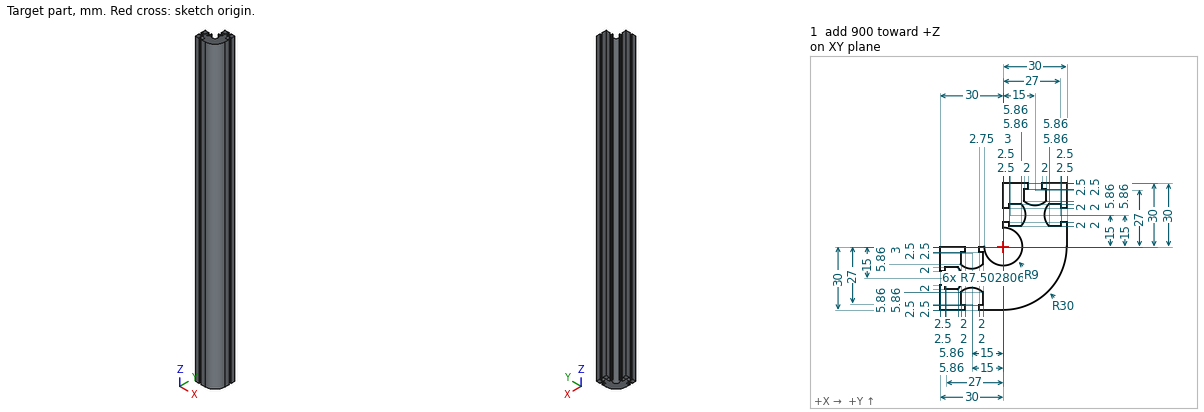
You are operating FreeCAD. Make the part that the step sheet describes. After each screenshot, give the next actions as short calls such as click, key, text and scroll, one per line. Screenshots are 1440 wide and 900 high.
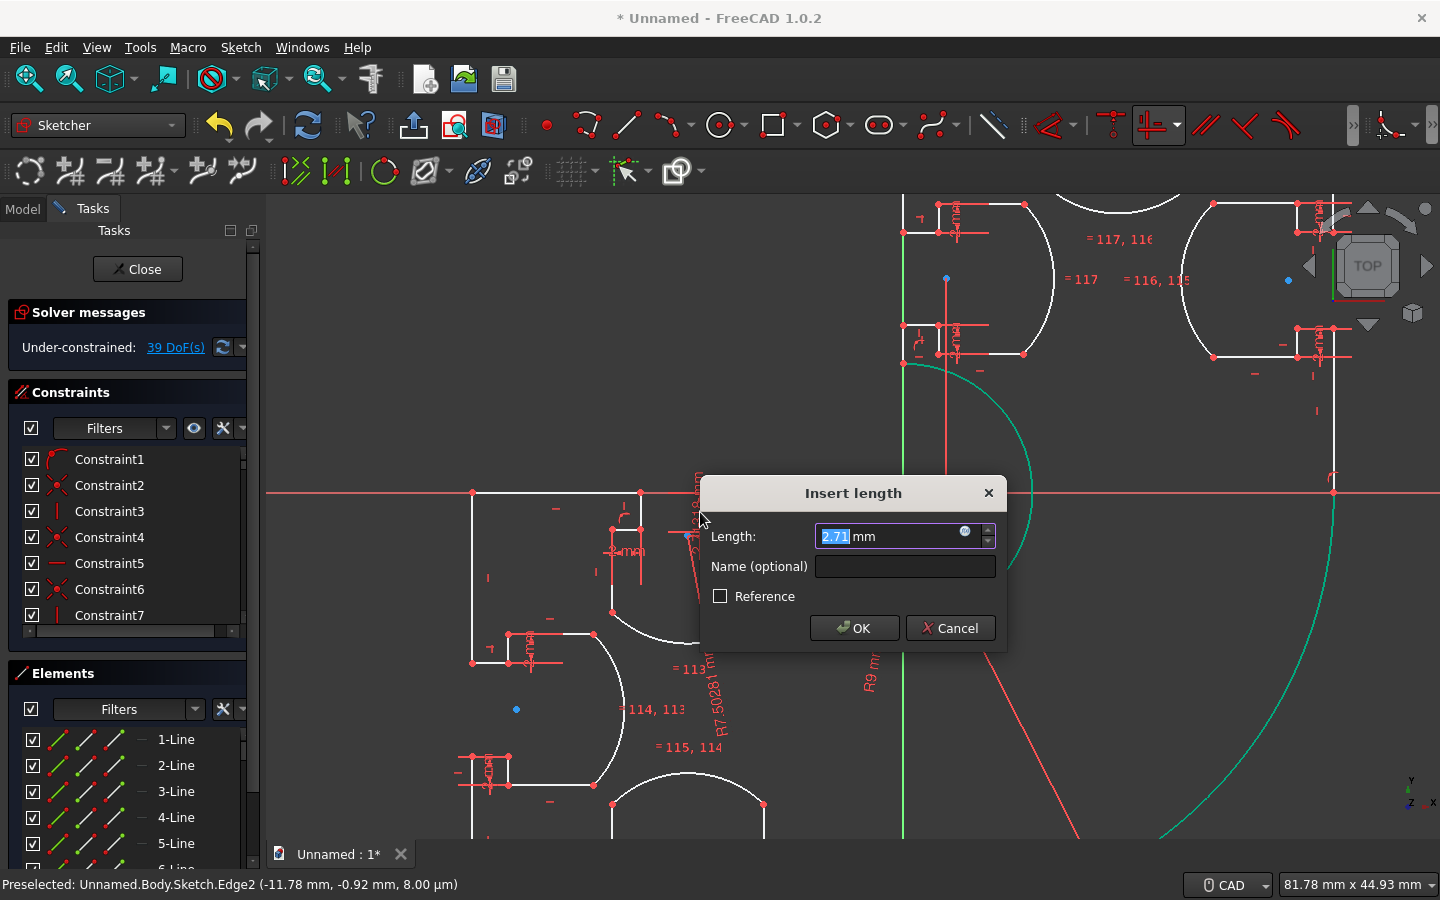
text(2.5)
key(Return)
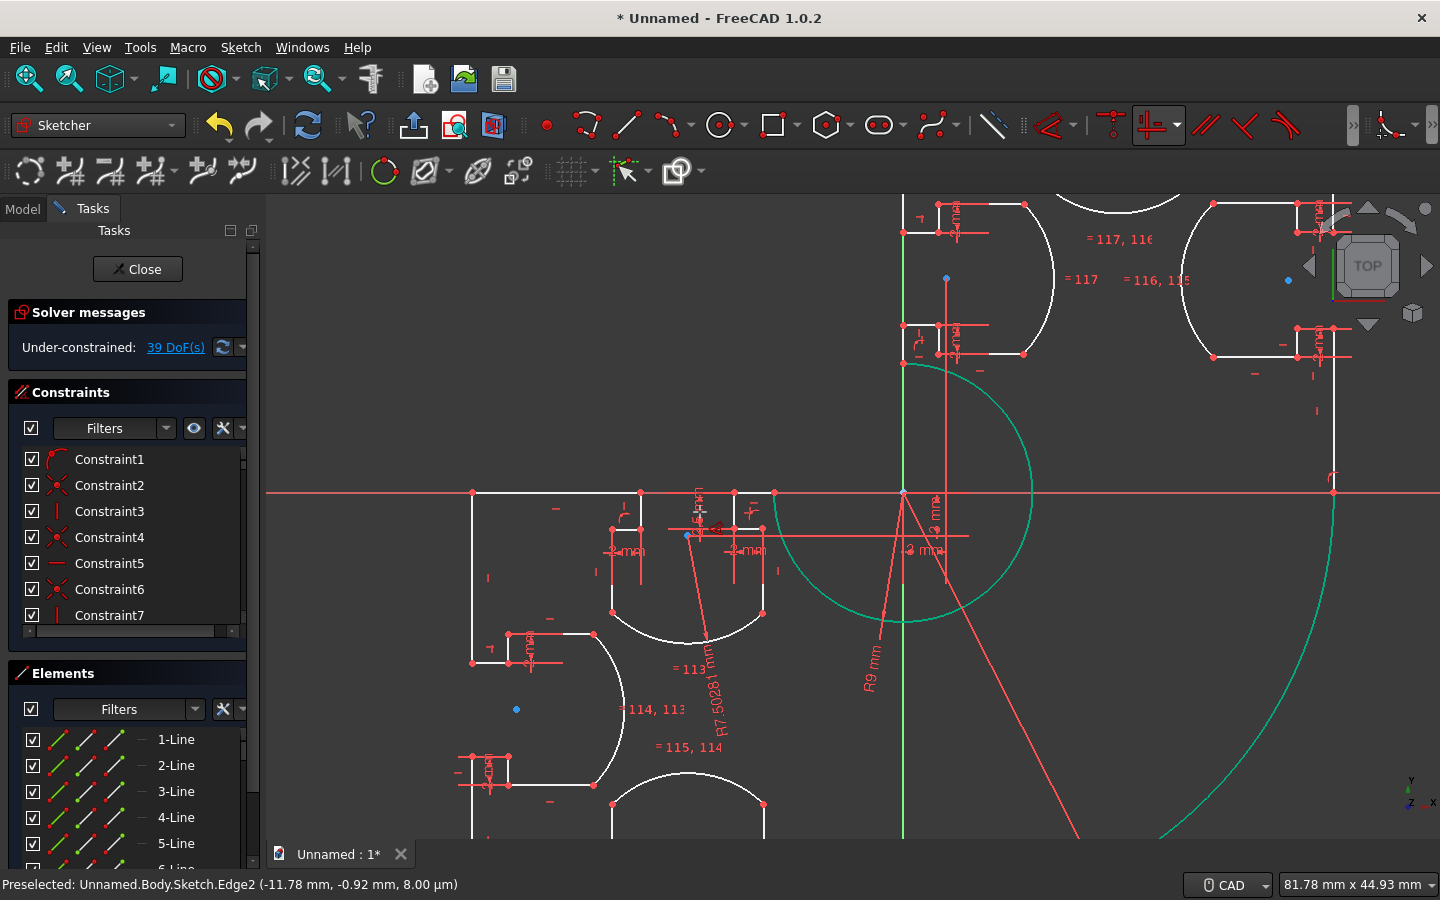
scroll(641, 519, up, 2)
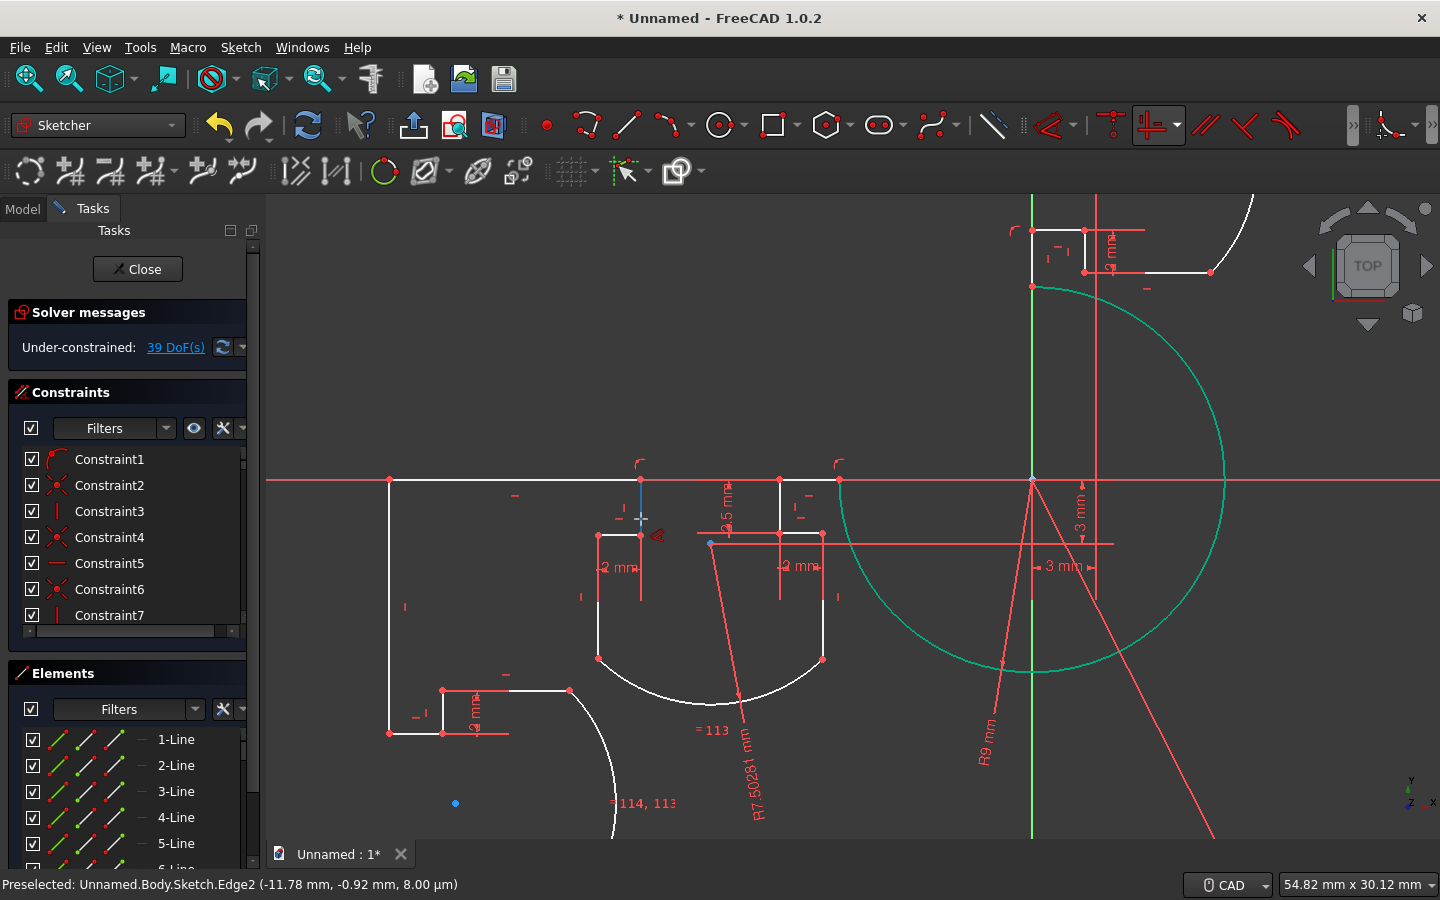
click(641, 518)
click(607, 507)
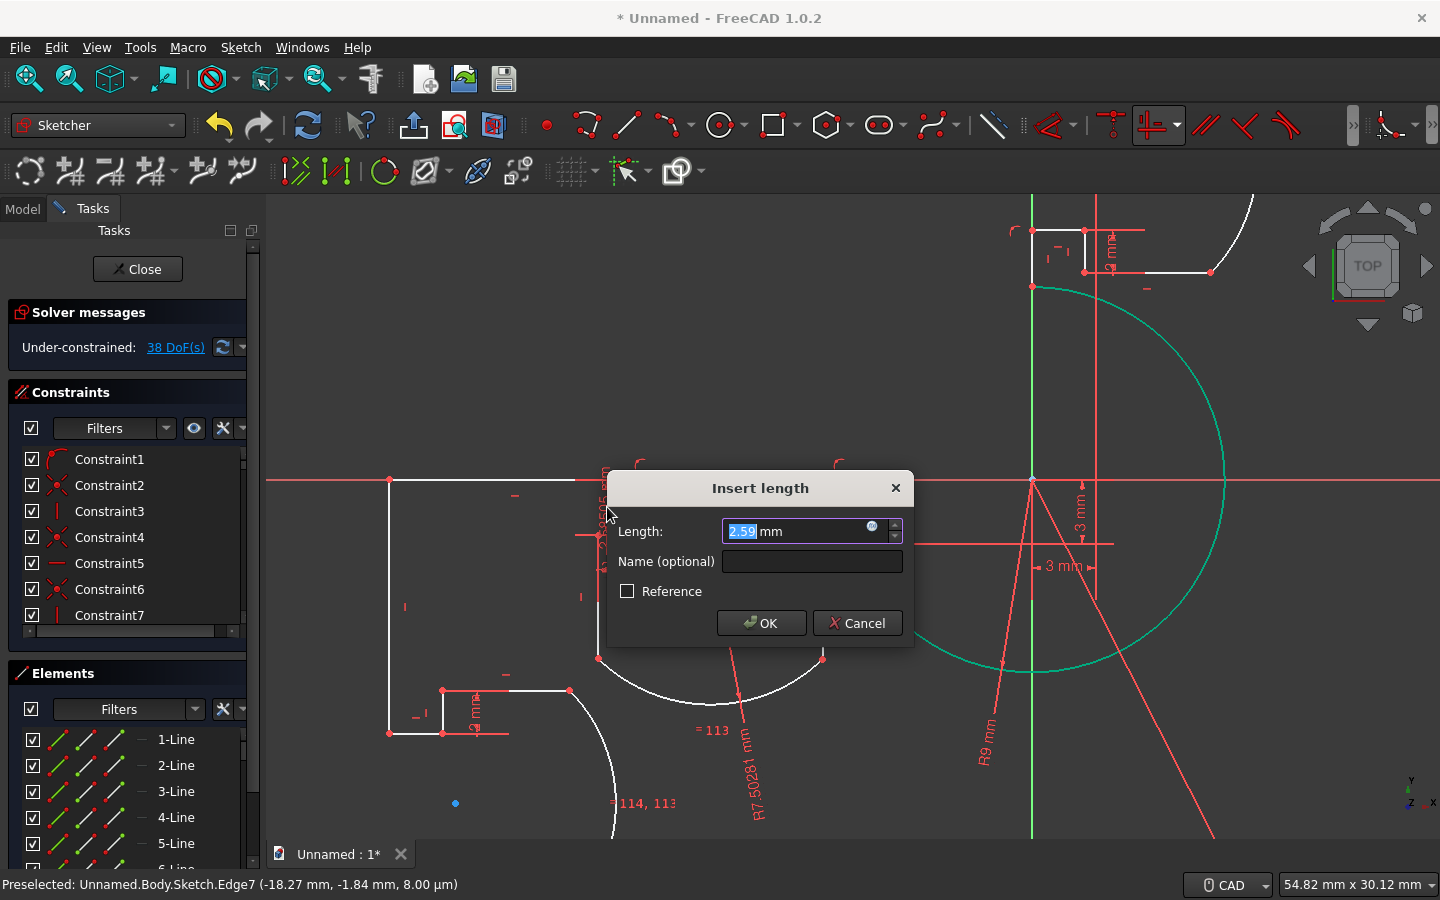
text(2.5)
key(Return)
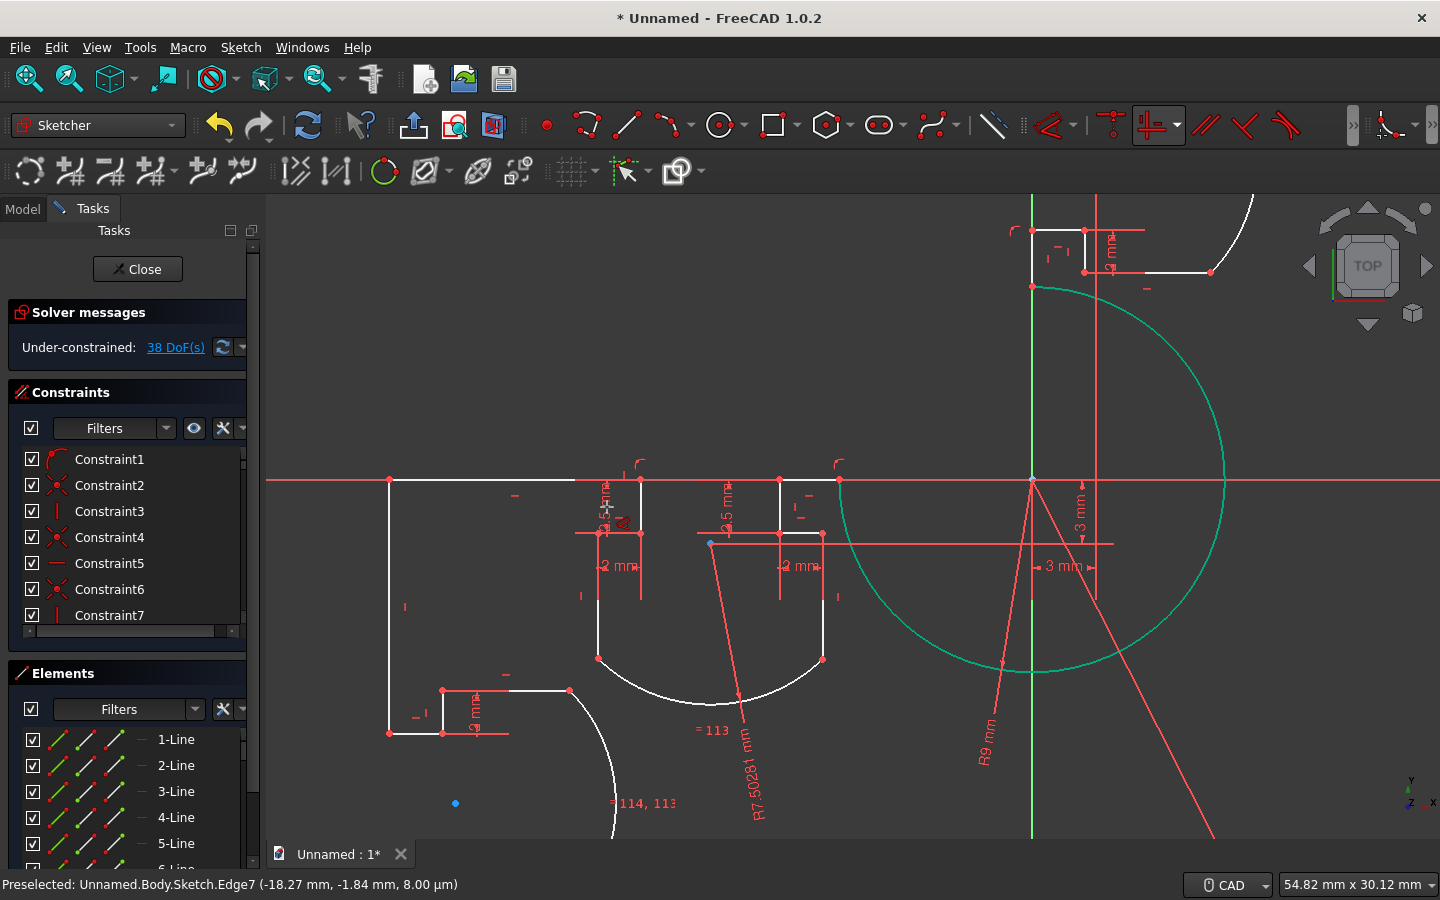
click(405, 734)
click(416, 768)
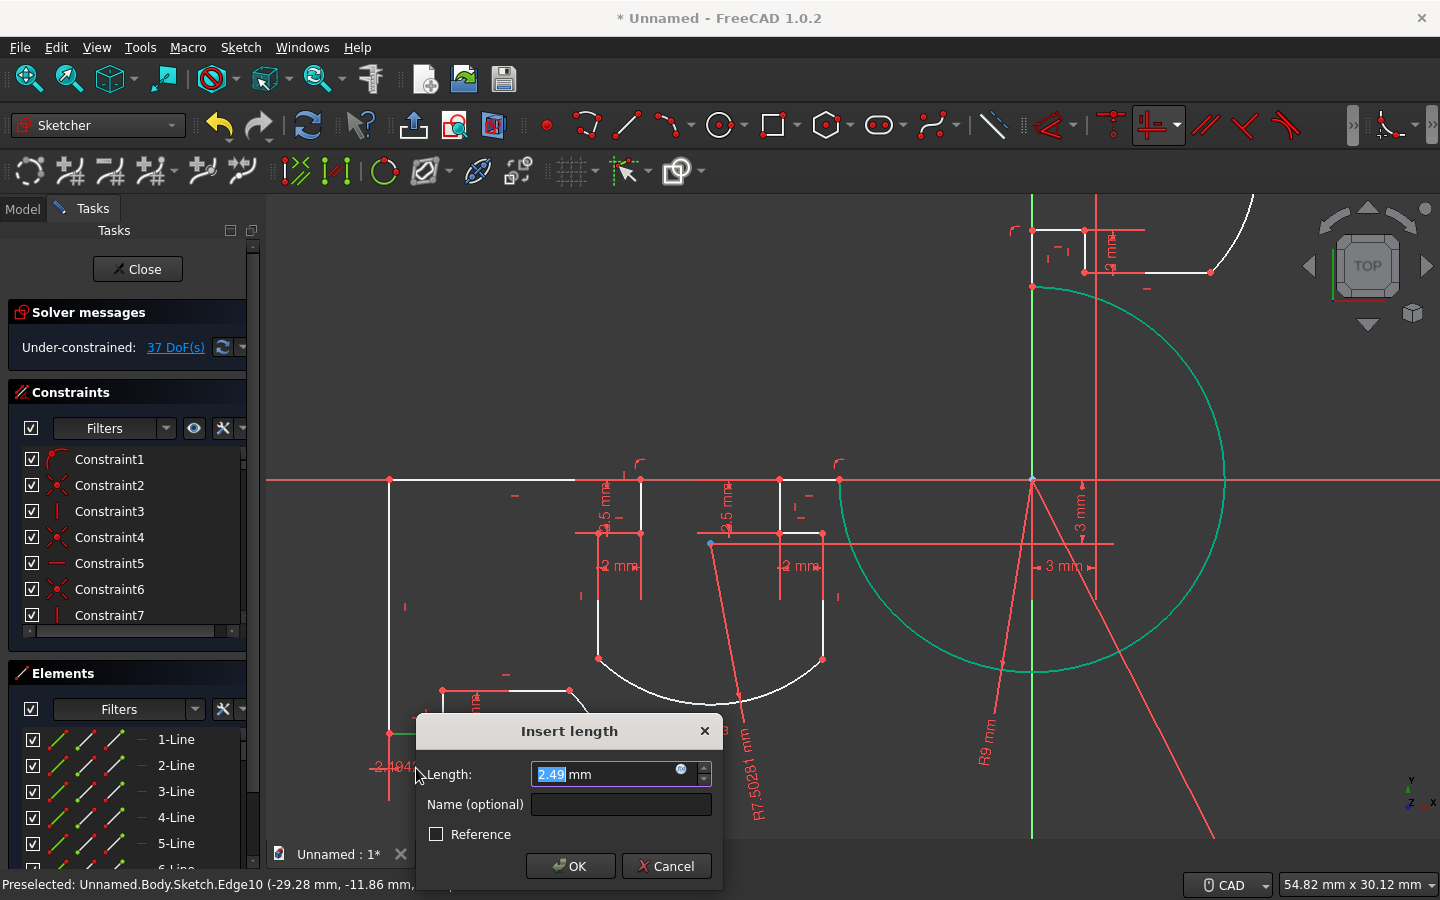
text(2.5)
key(Return)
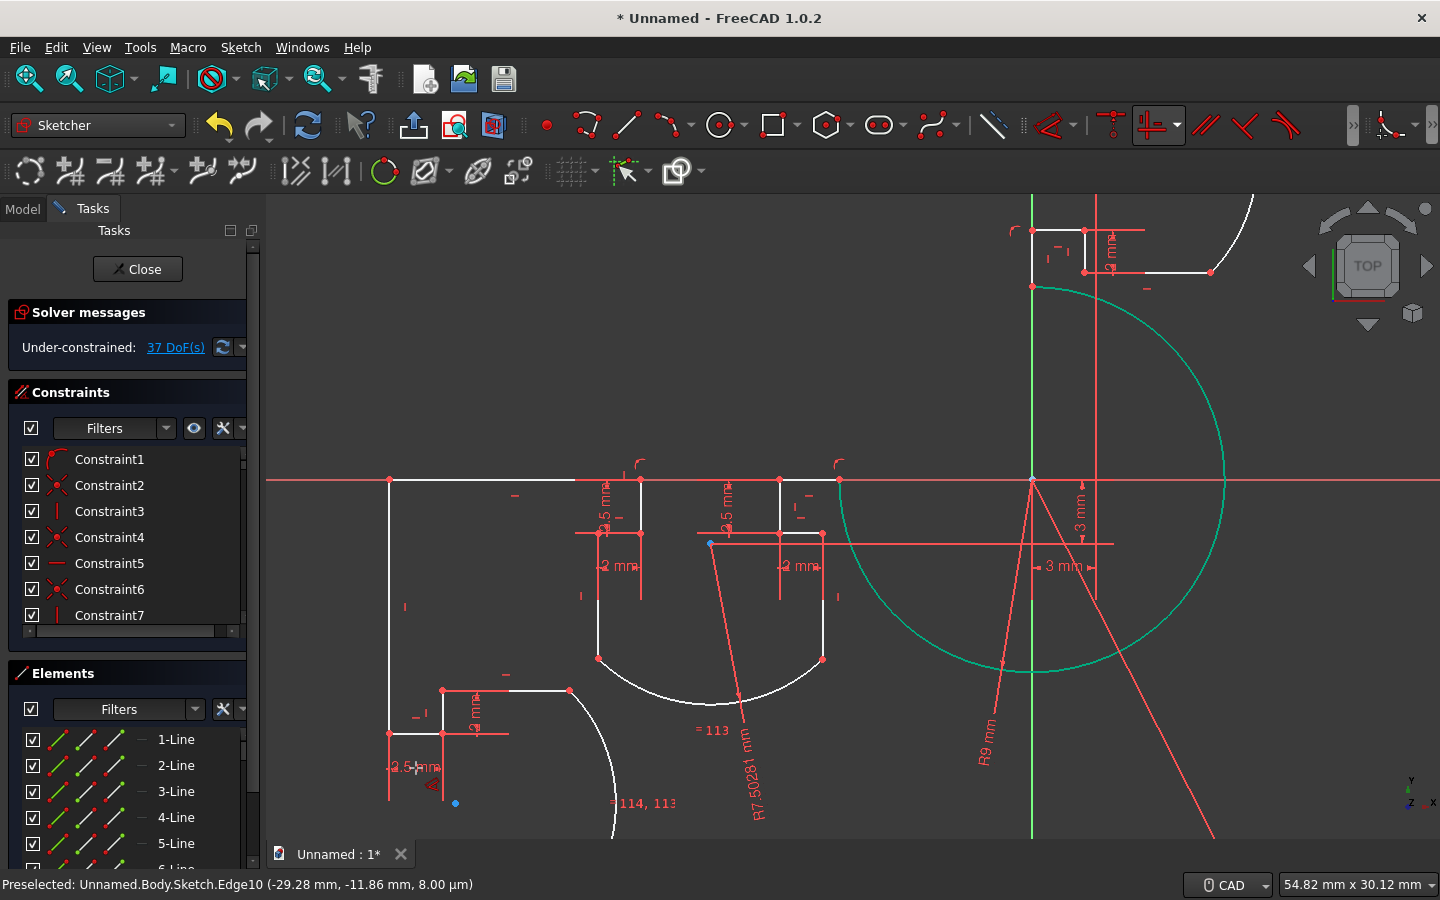
scroll(678, 532, down, 6)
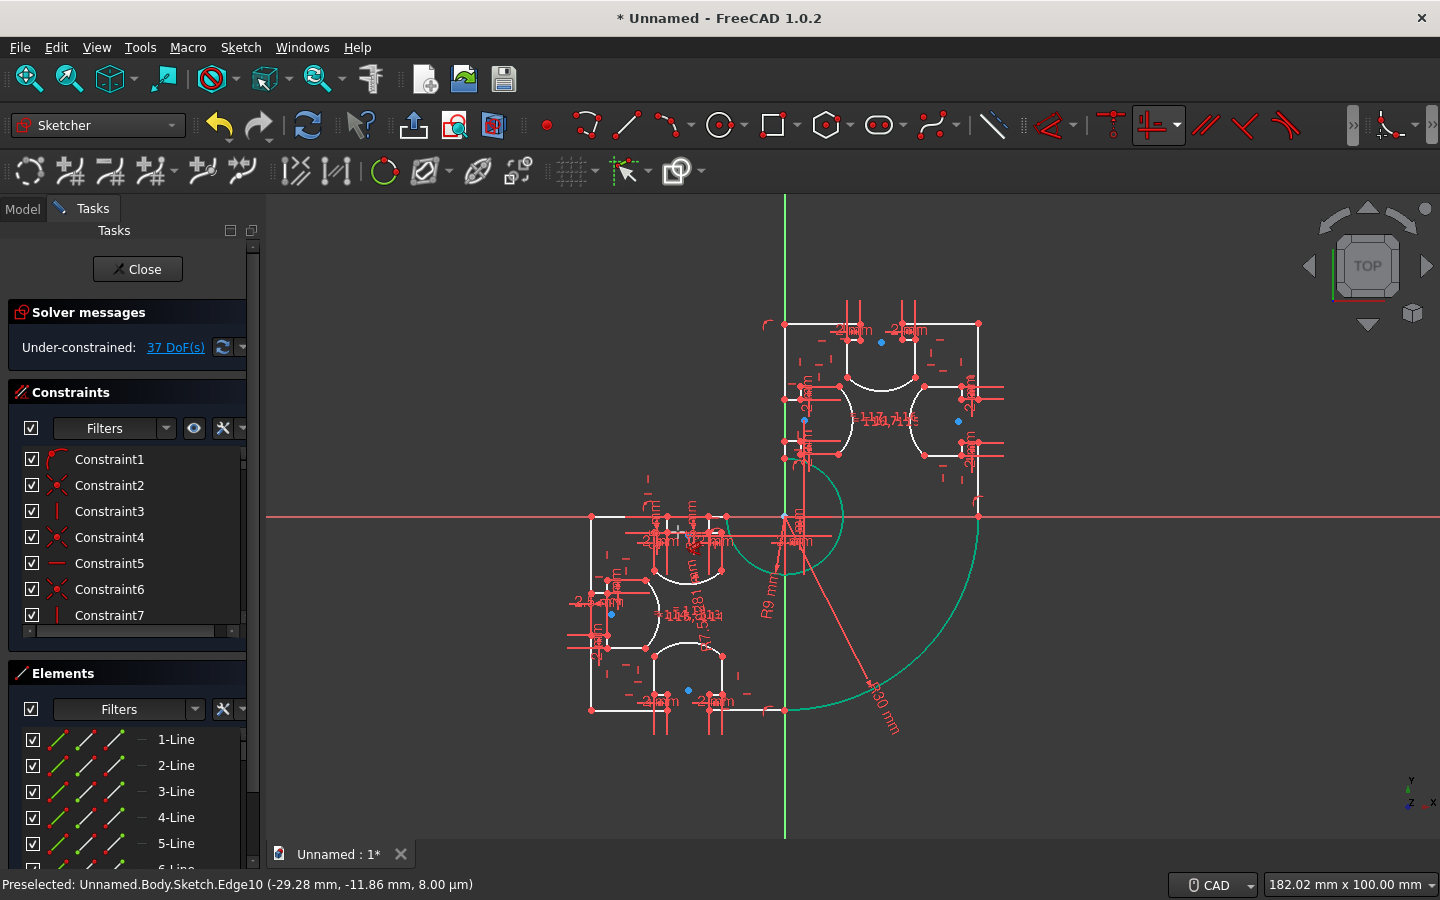
scroll(603, 635, up, 6)